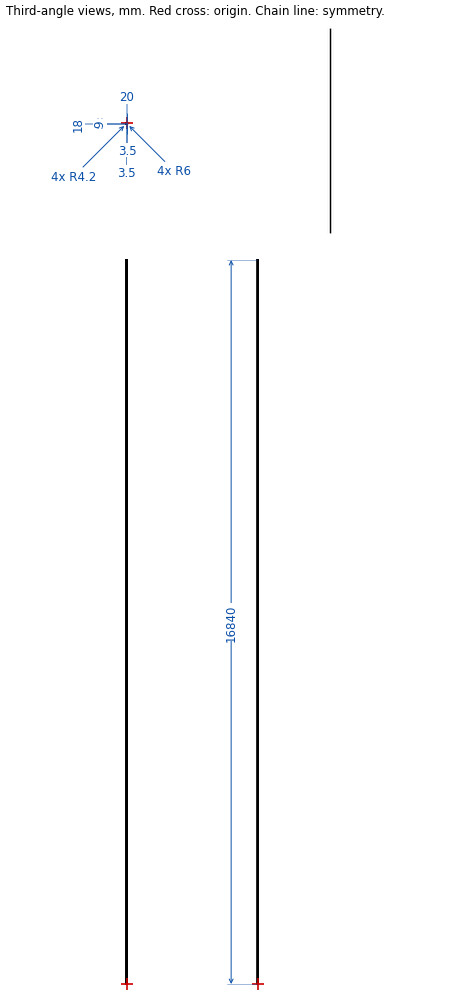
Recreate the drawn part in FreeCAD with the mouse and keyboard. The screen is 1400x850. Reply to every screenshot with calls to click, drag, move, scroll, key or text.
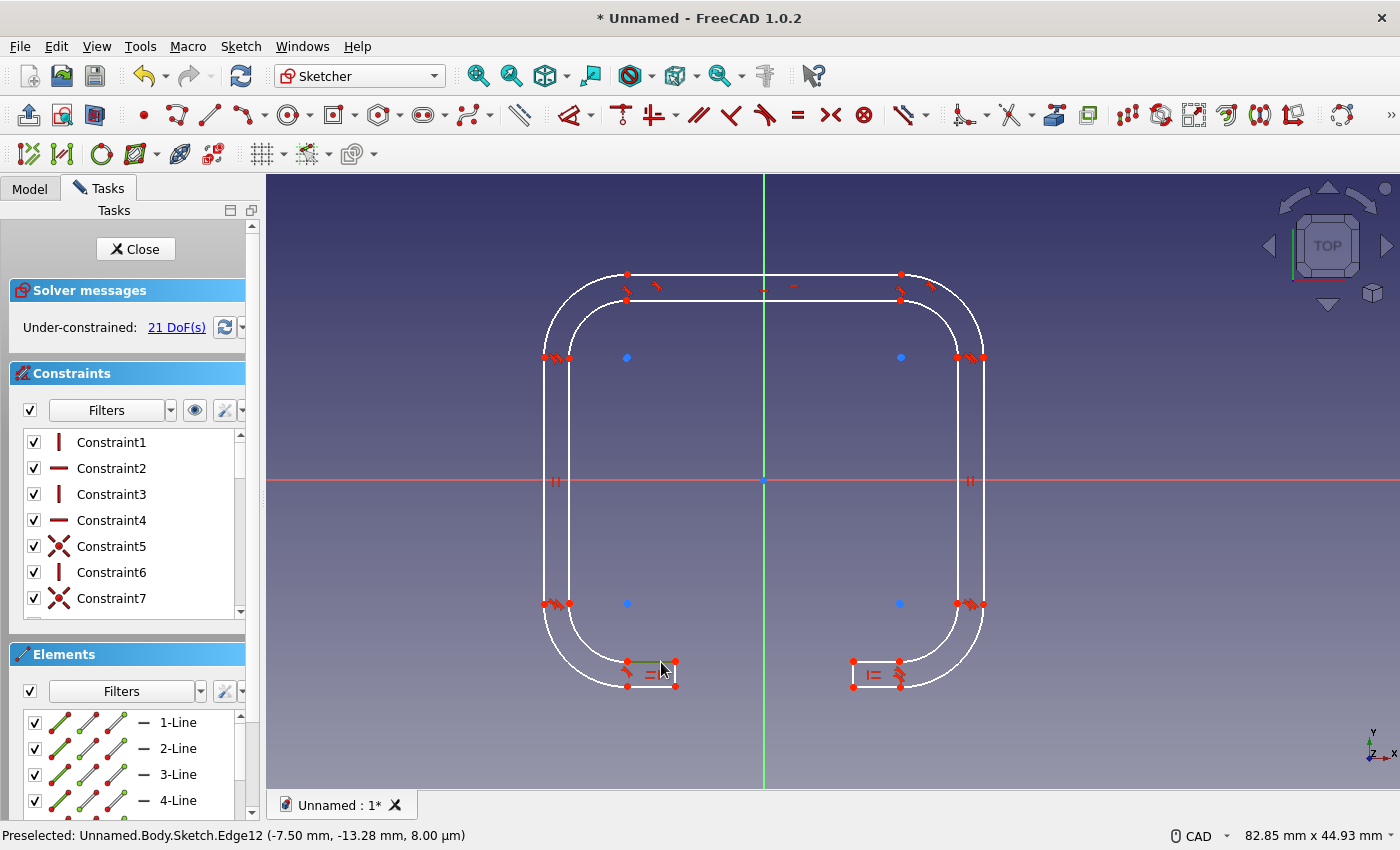
click(575, 630)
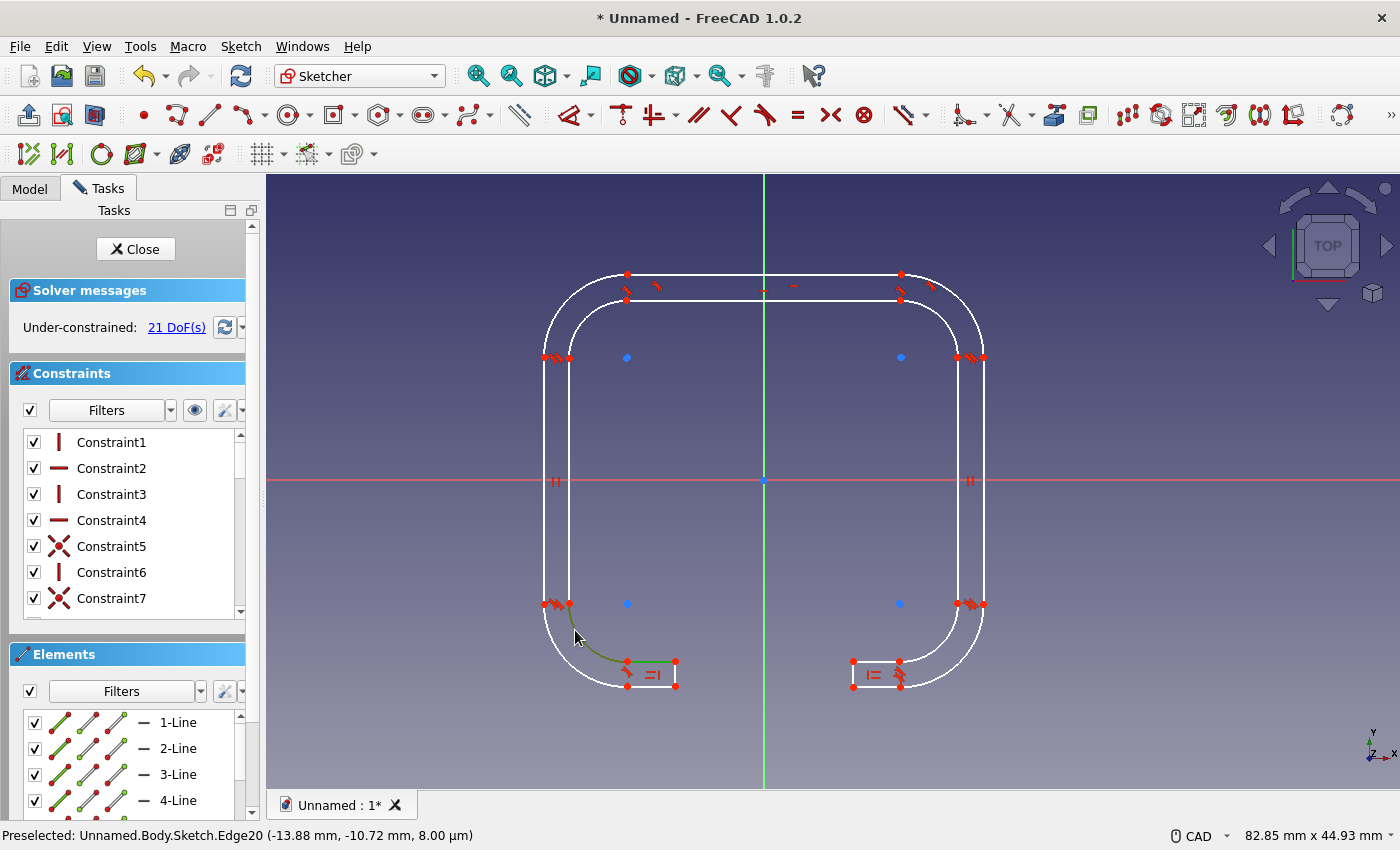
click(765, 116)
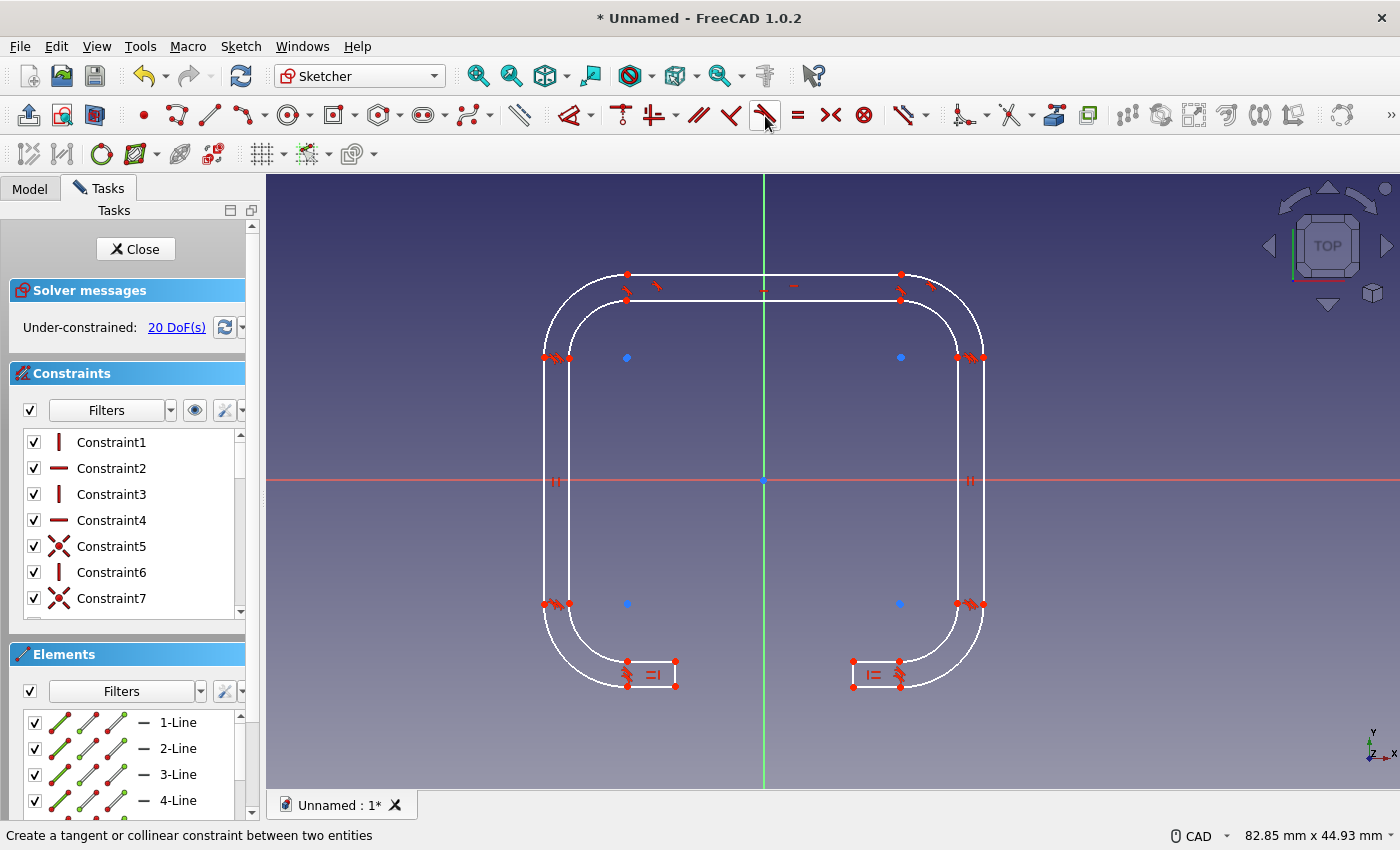
click(926, 656)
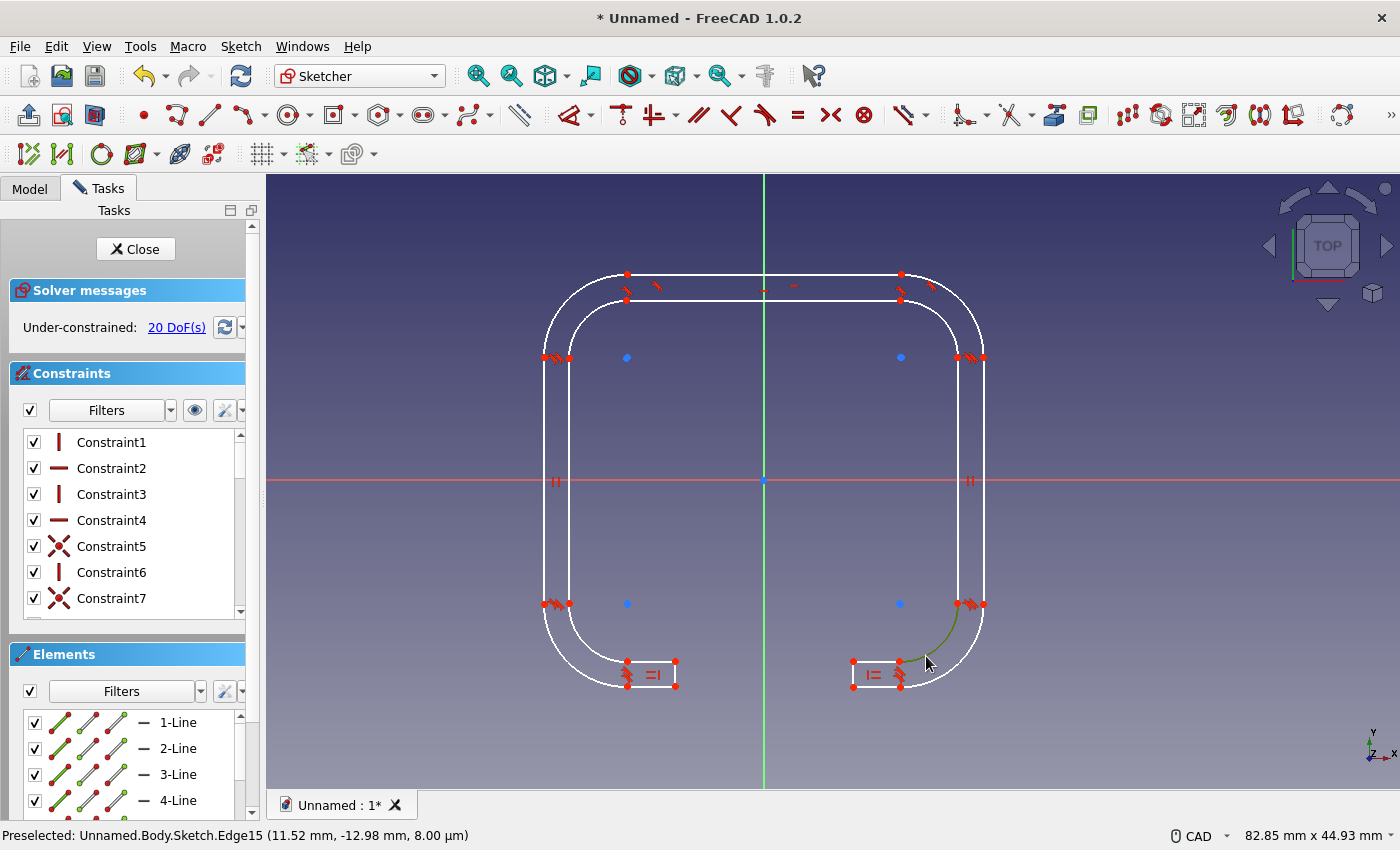
click(938, 678)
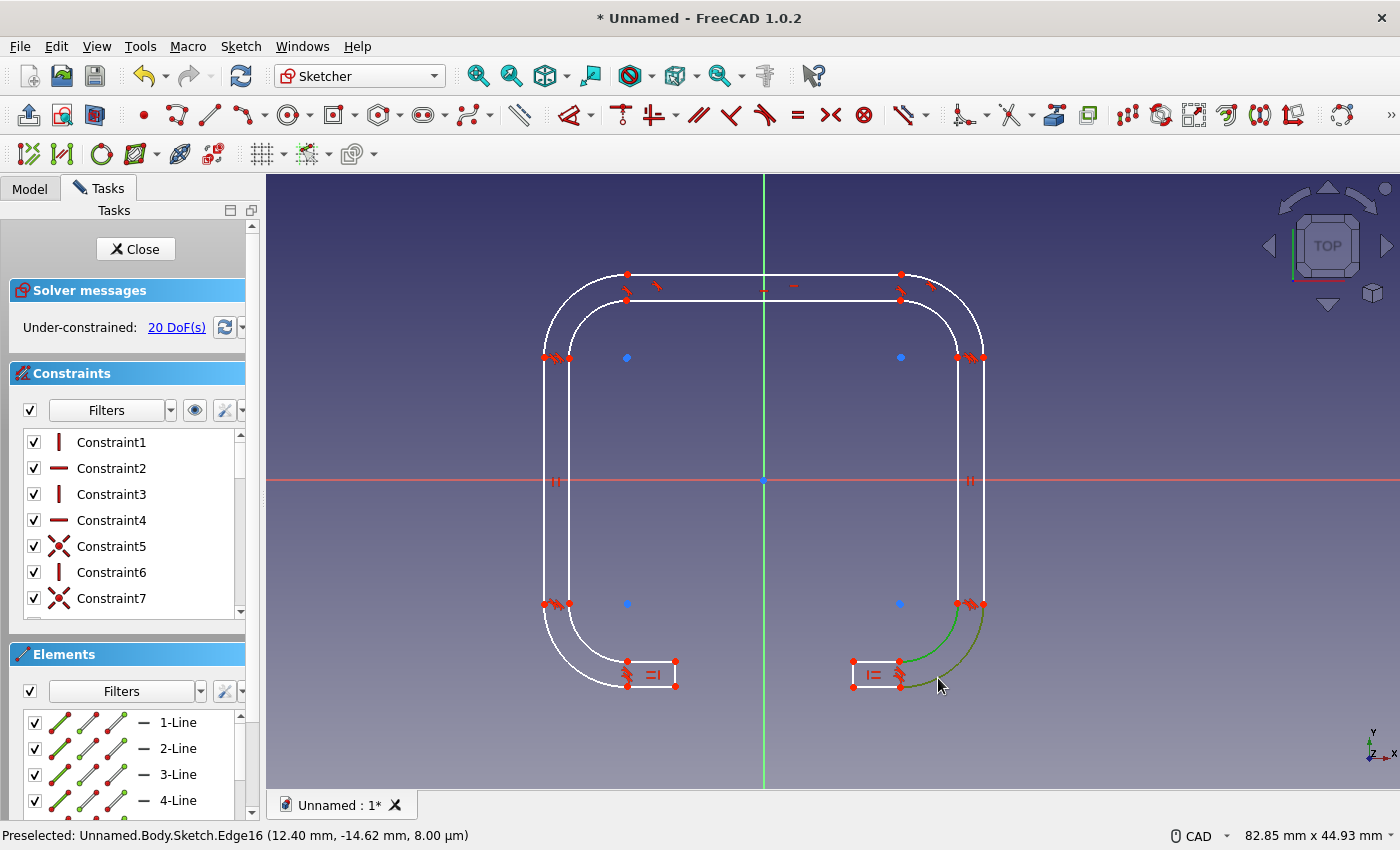
click(621, 116)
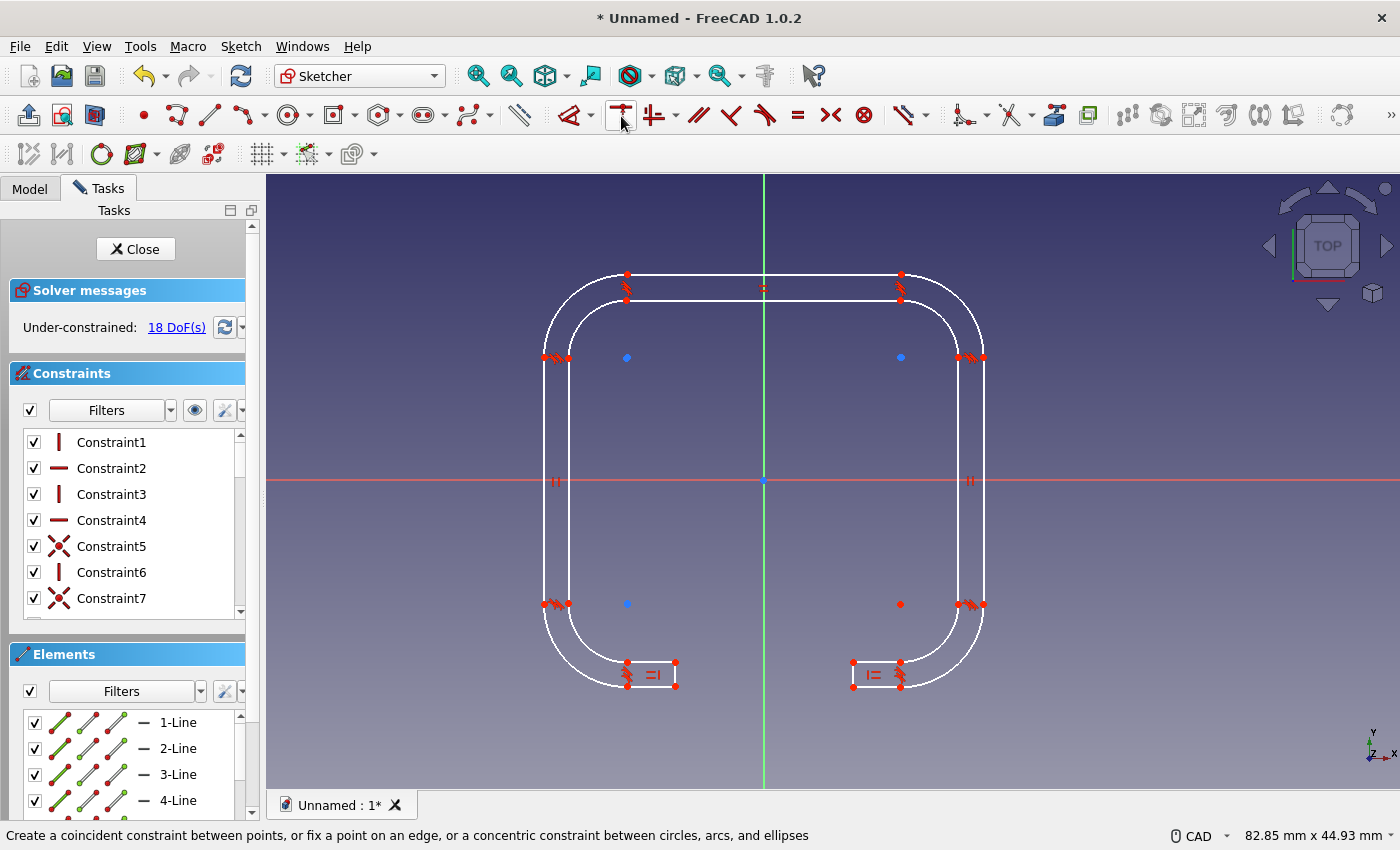
click(952, 332)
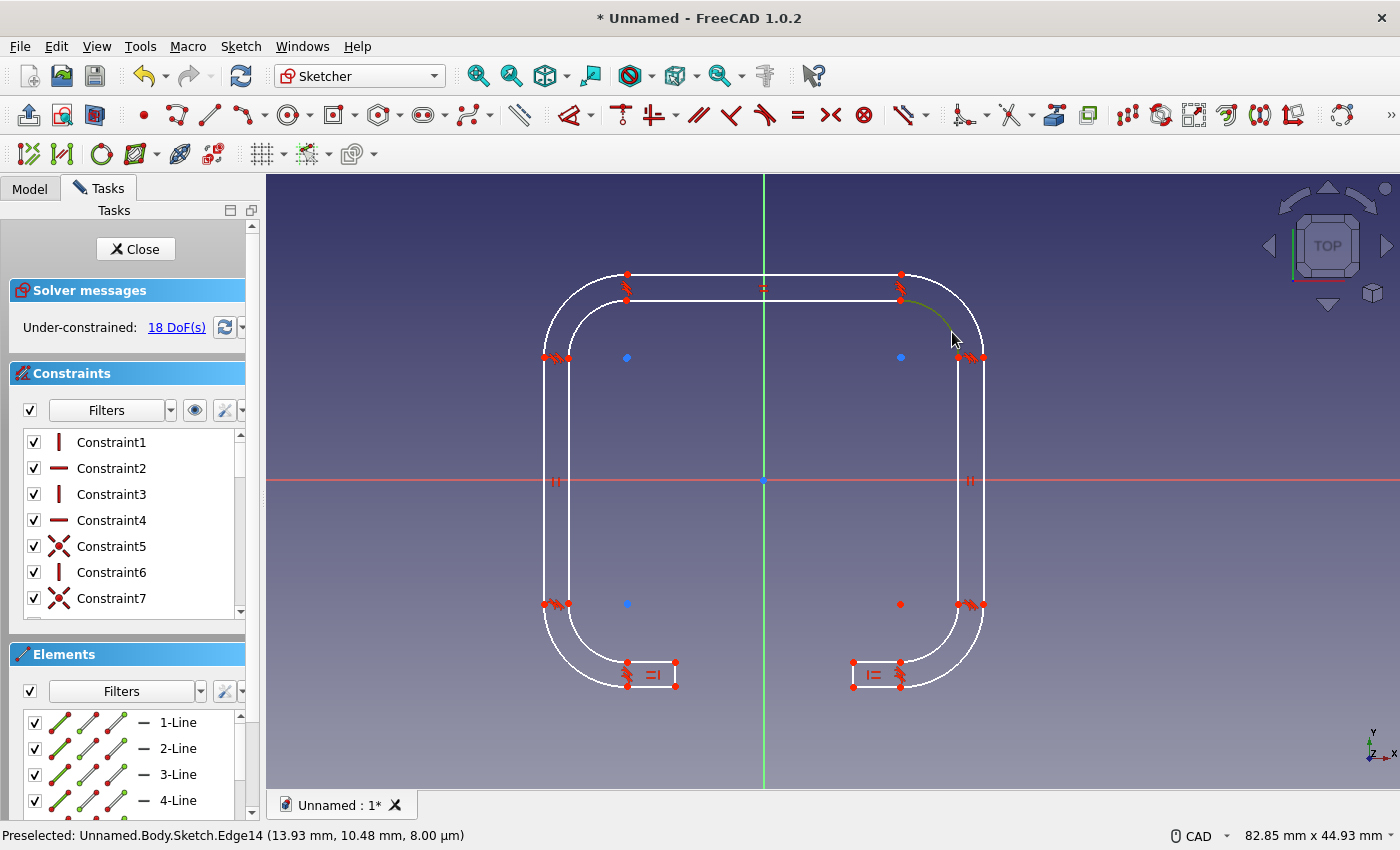
click(975, 320)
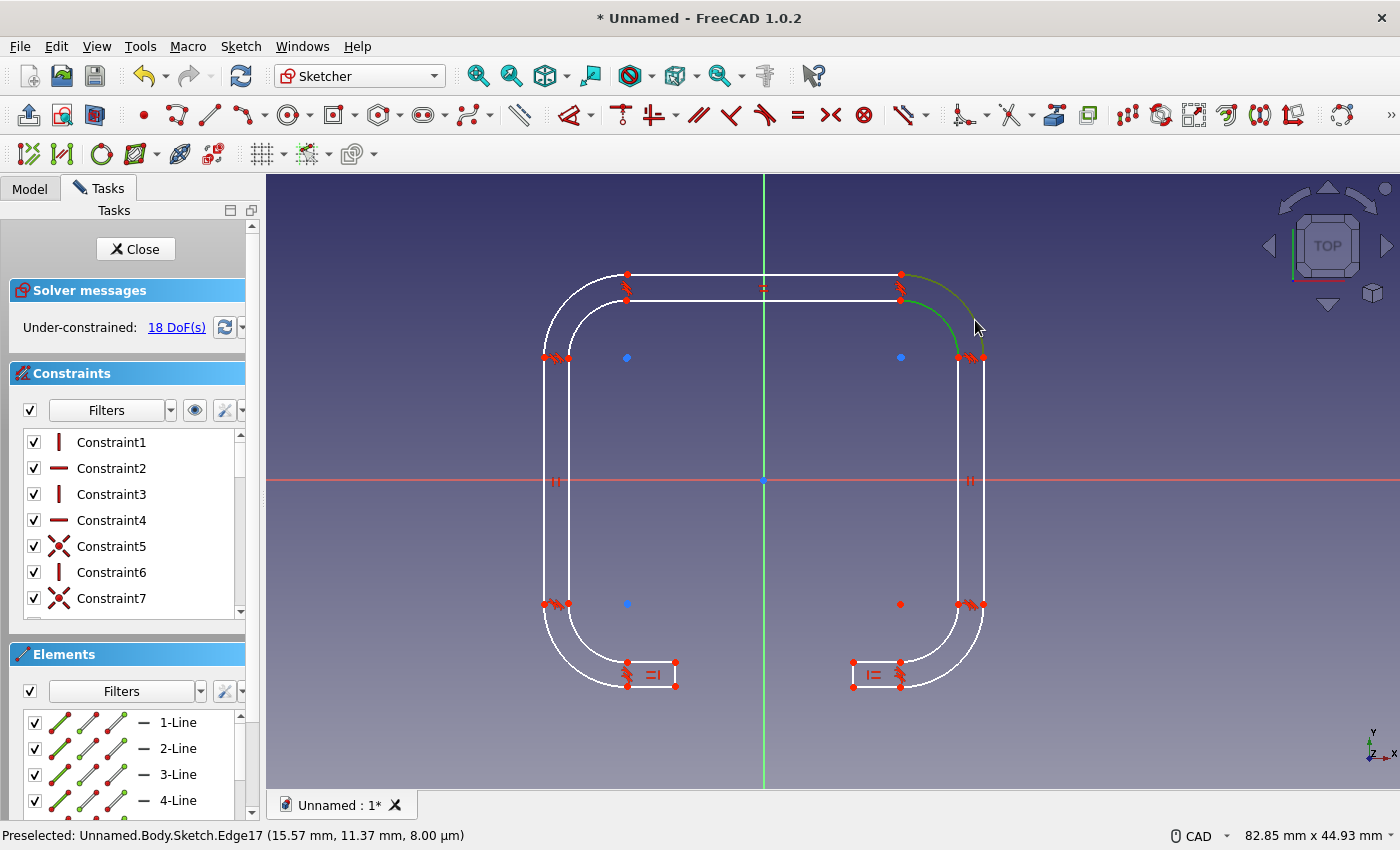
click(621, 116)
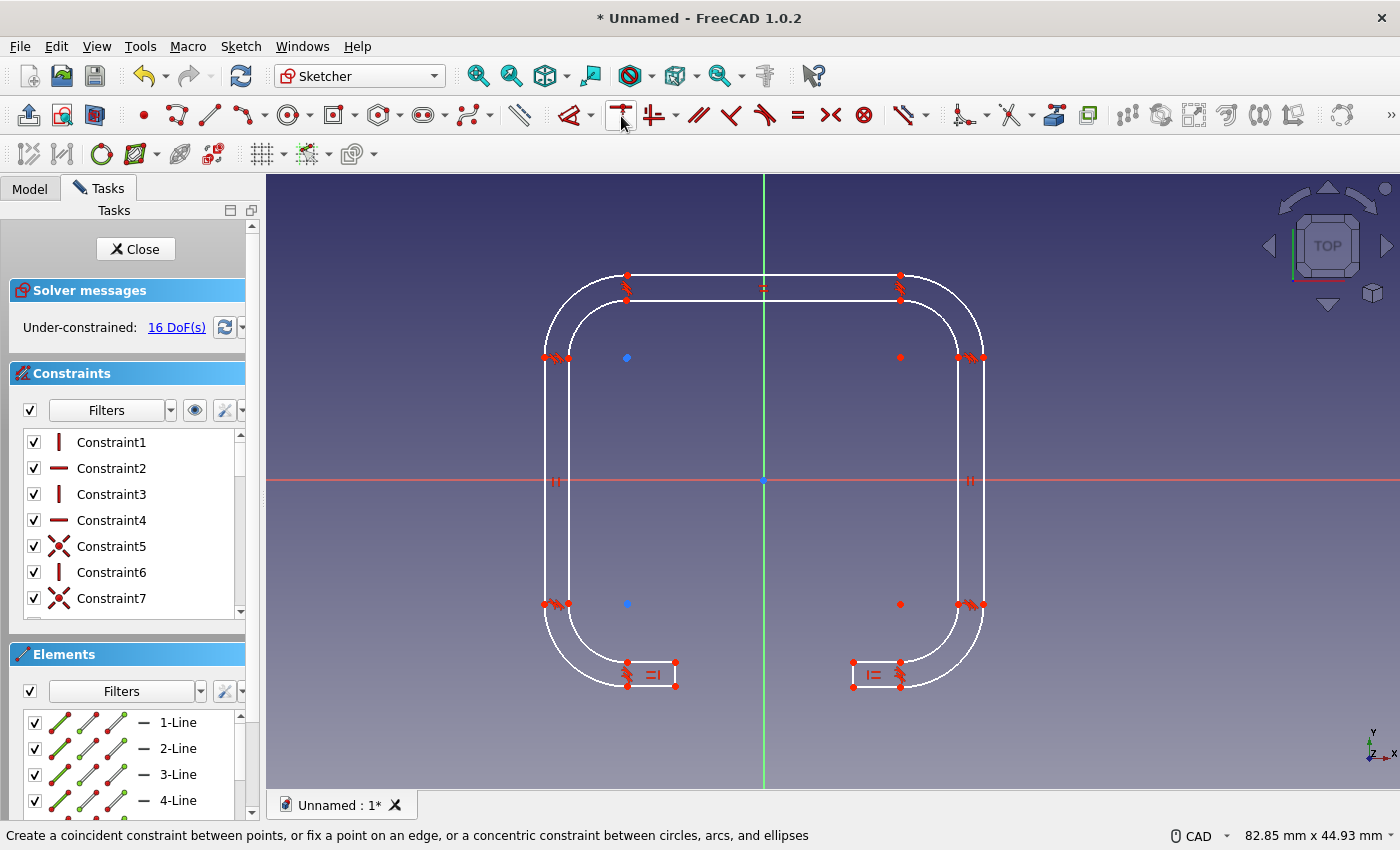
click(600, 307)